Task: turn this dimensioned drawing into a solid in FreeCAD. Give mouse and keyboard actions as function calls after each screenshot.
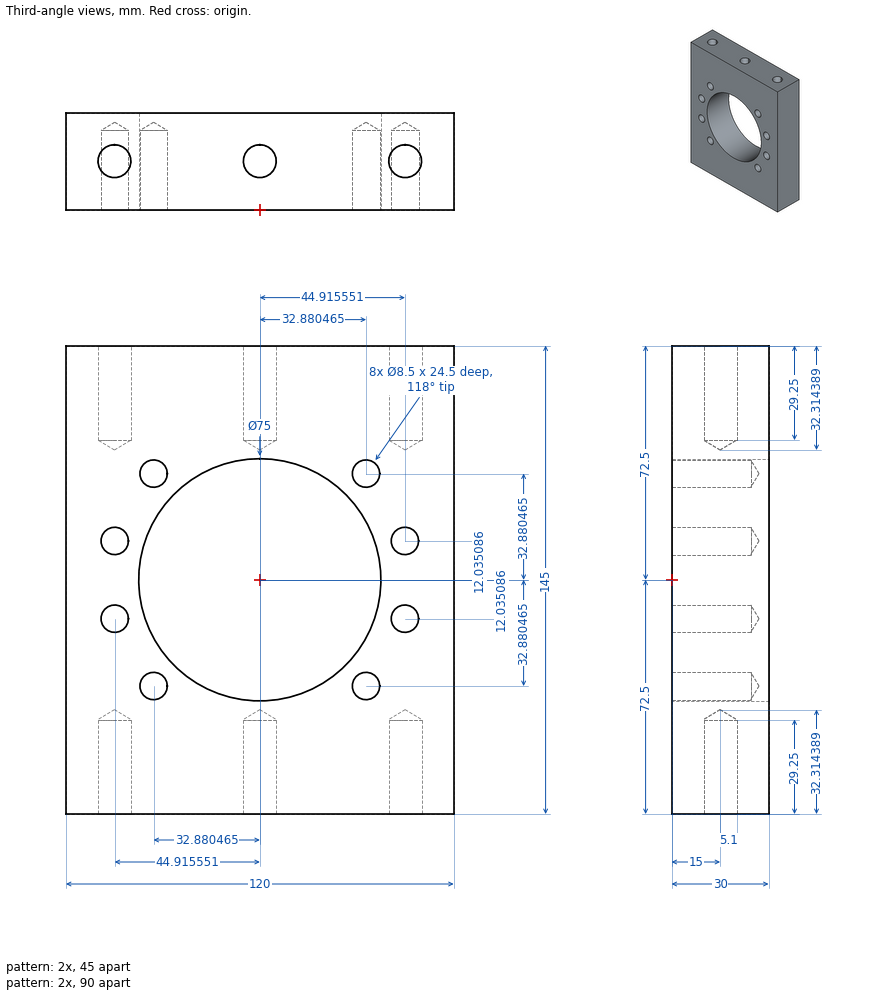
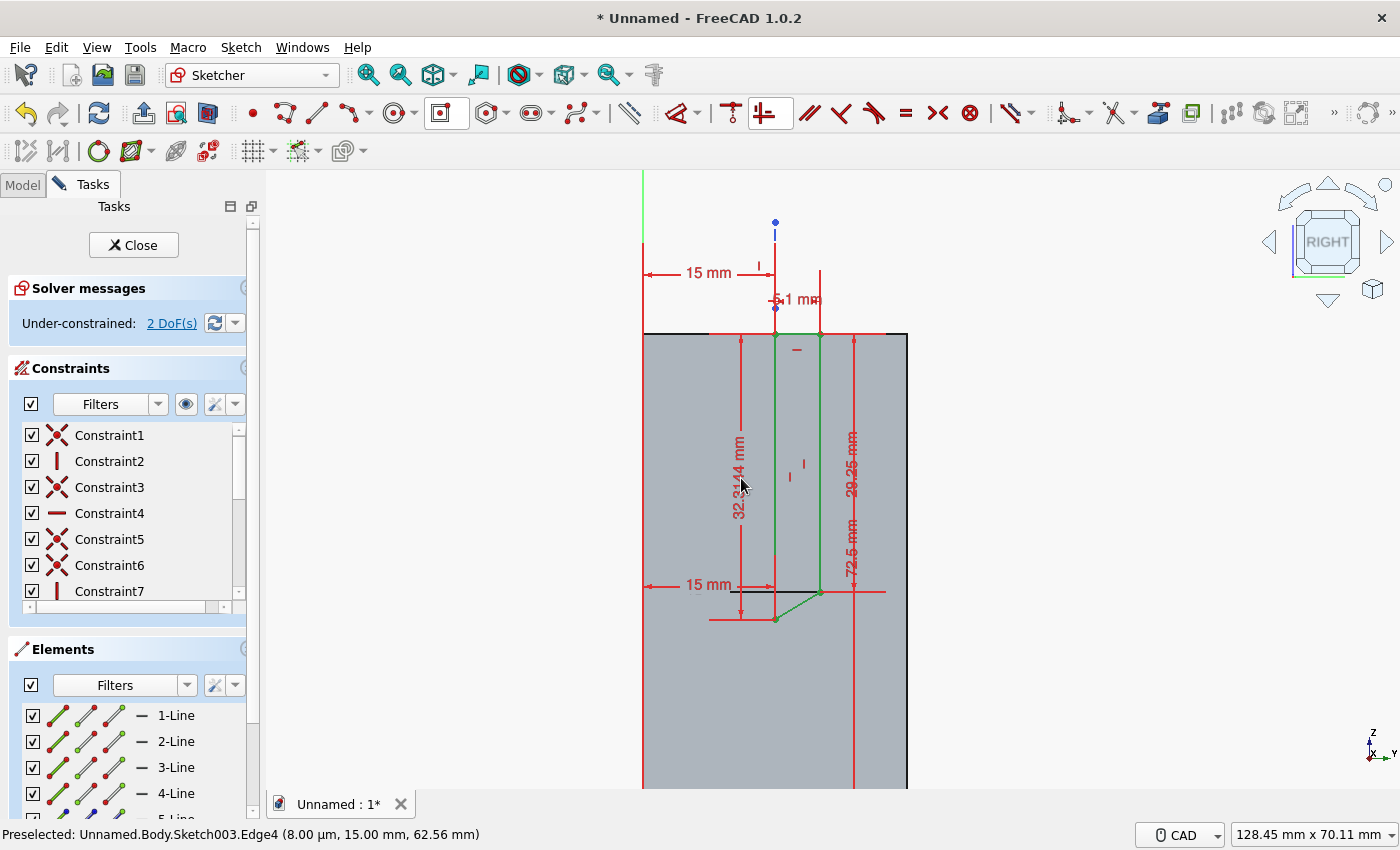
click(134, 245)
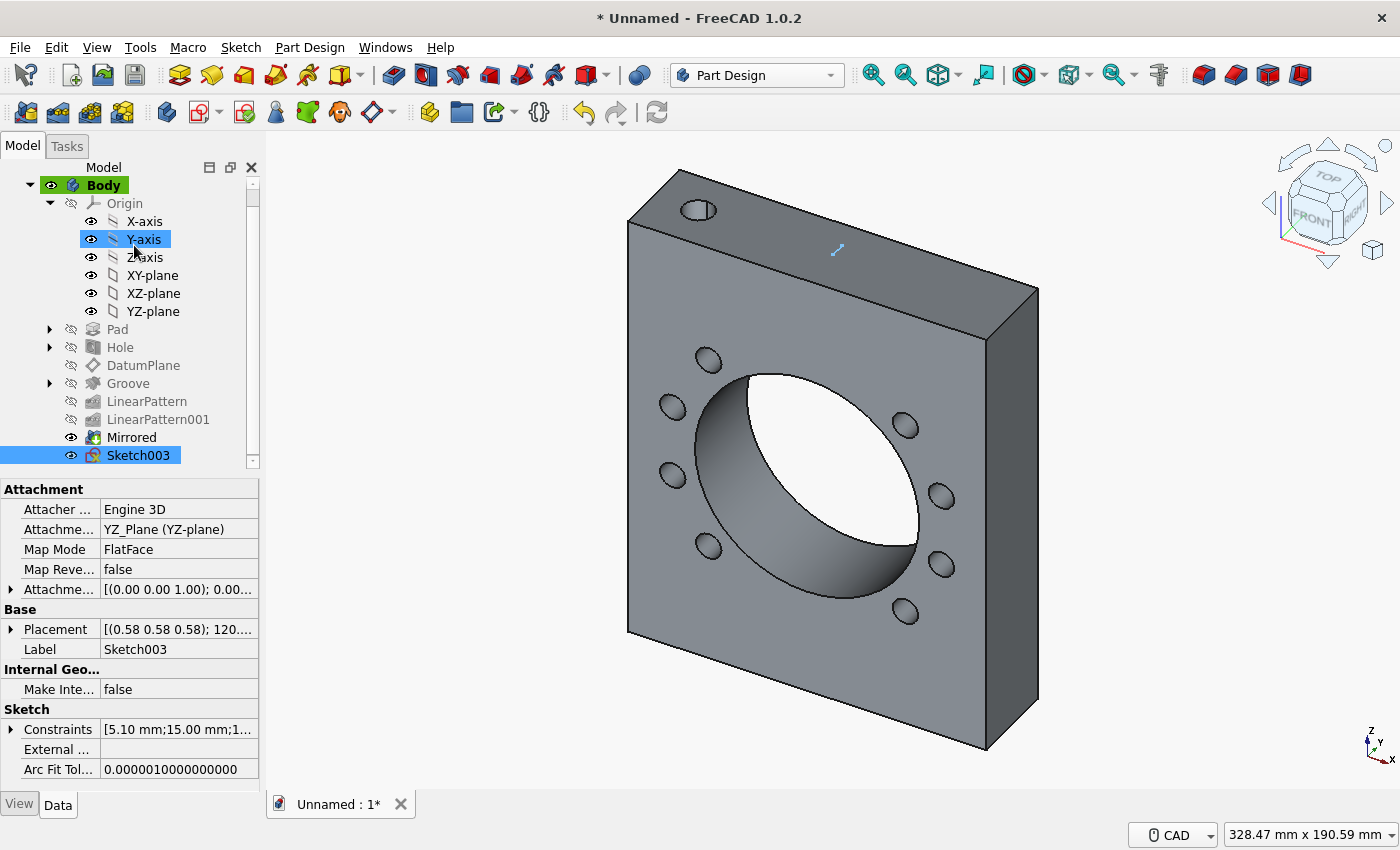
click(458, 76)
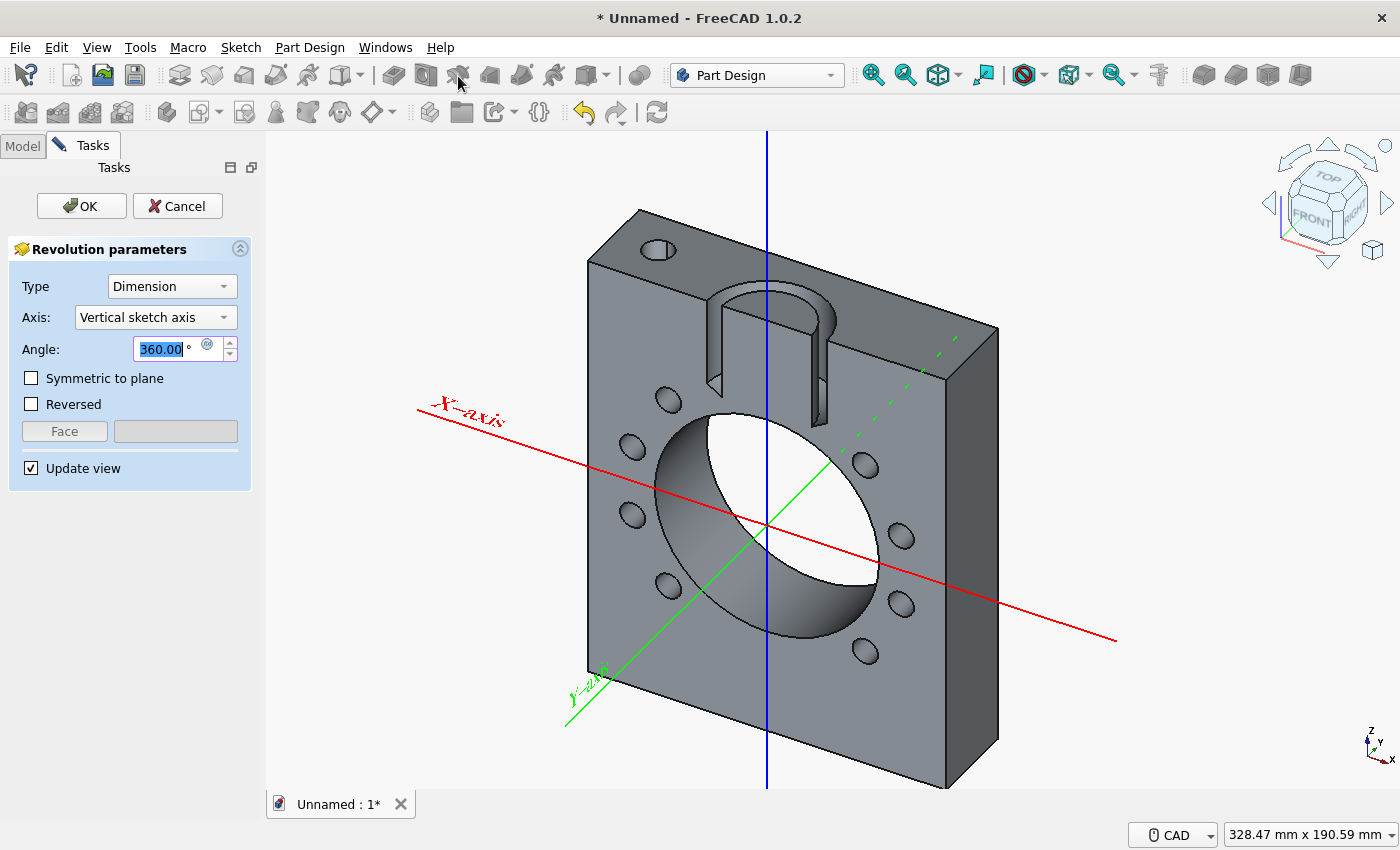
click(156, 318)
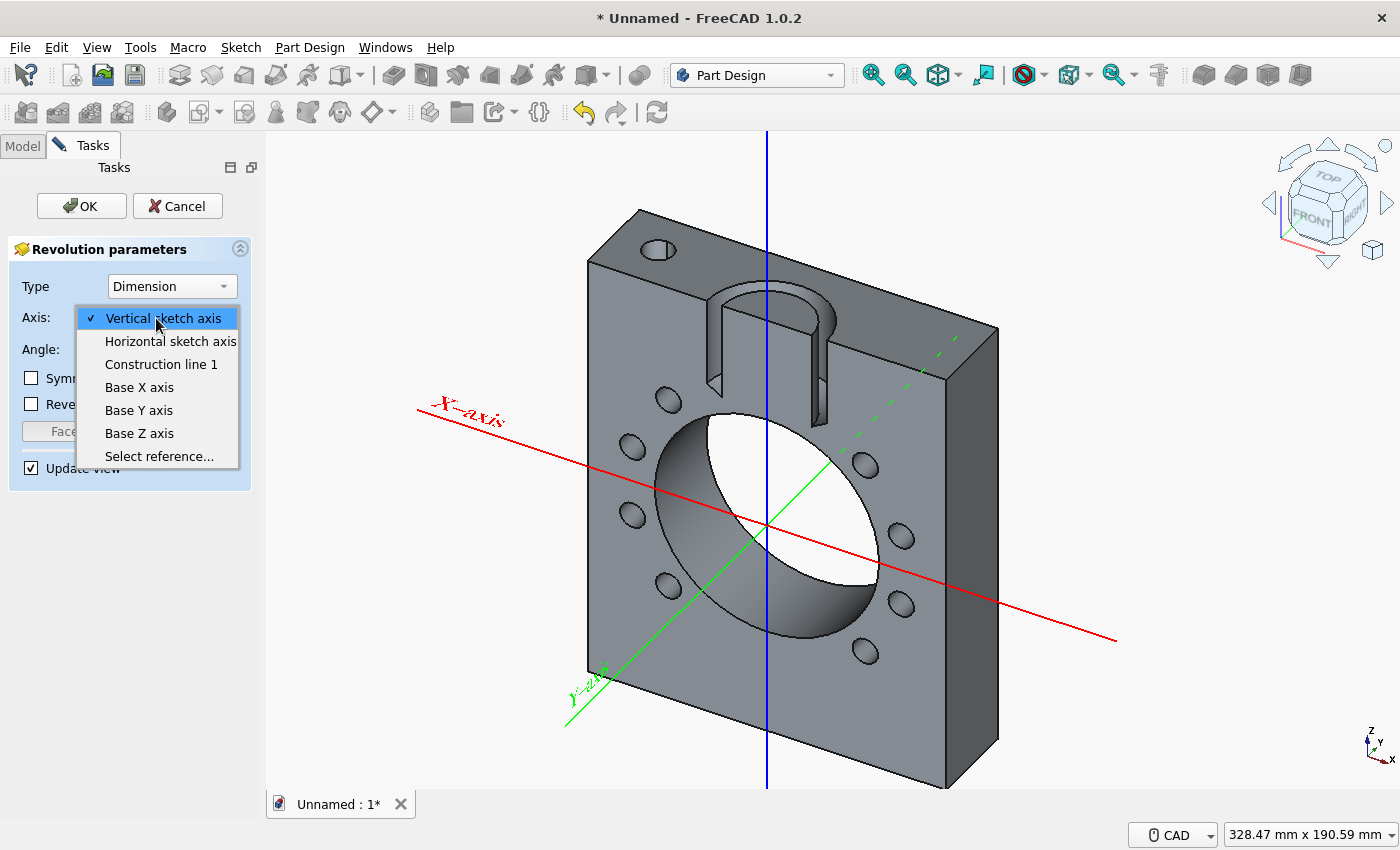
click(156, 364)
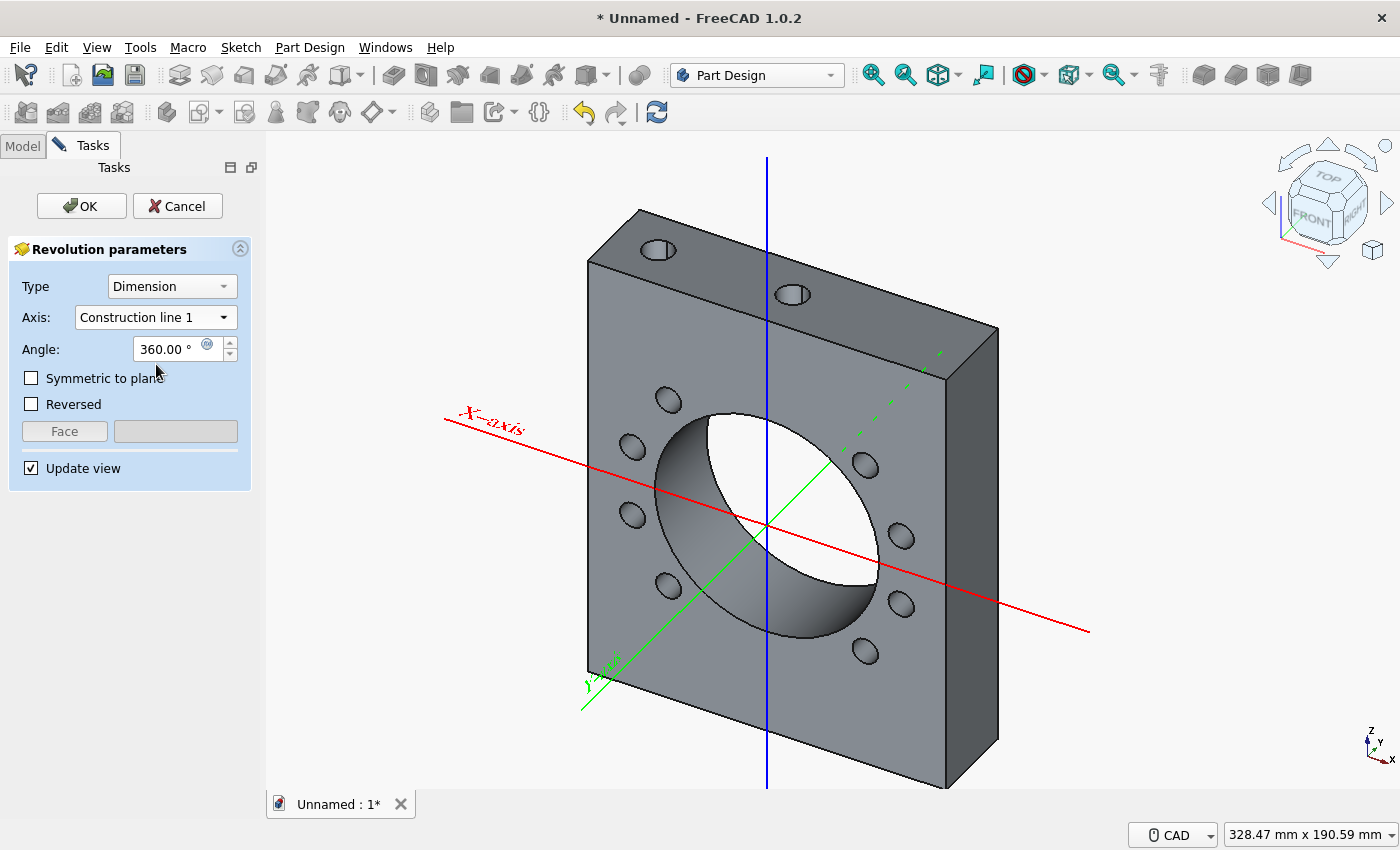
click(82, 206)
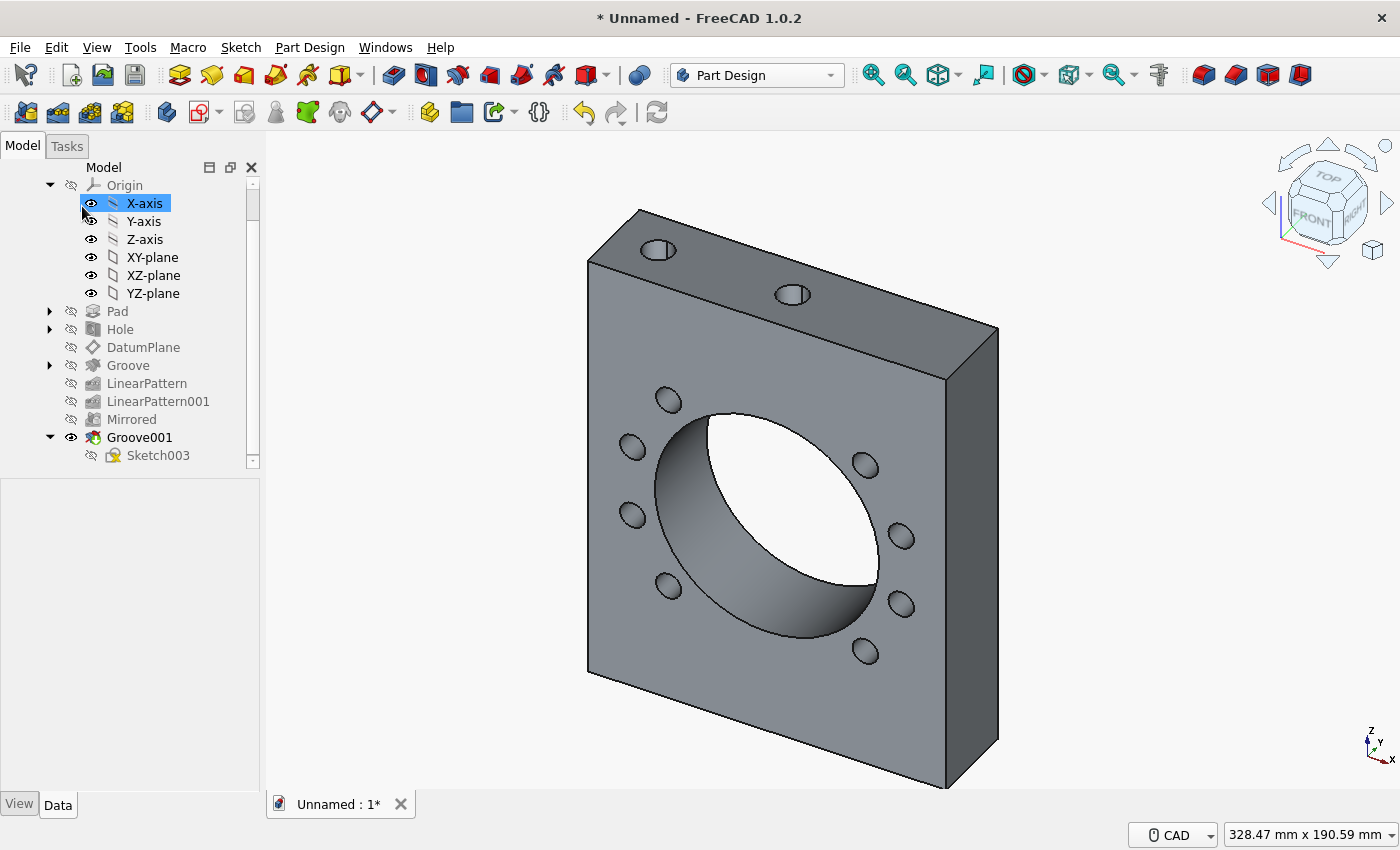
click(136, 293)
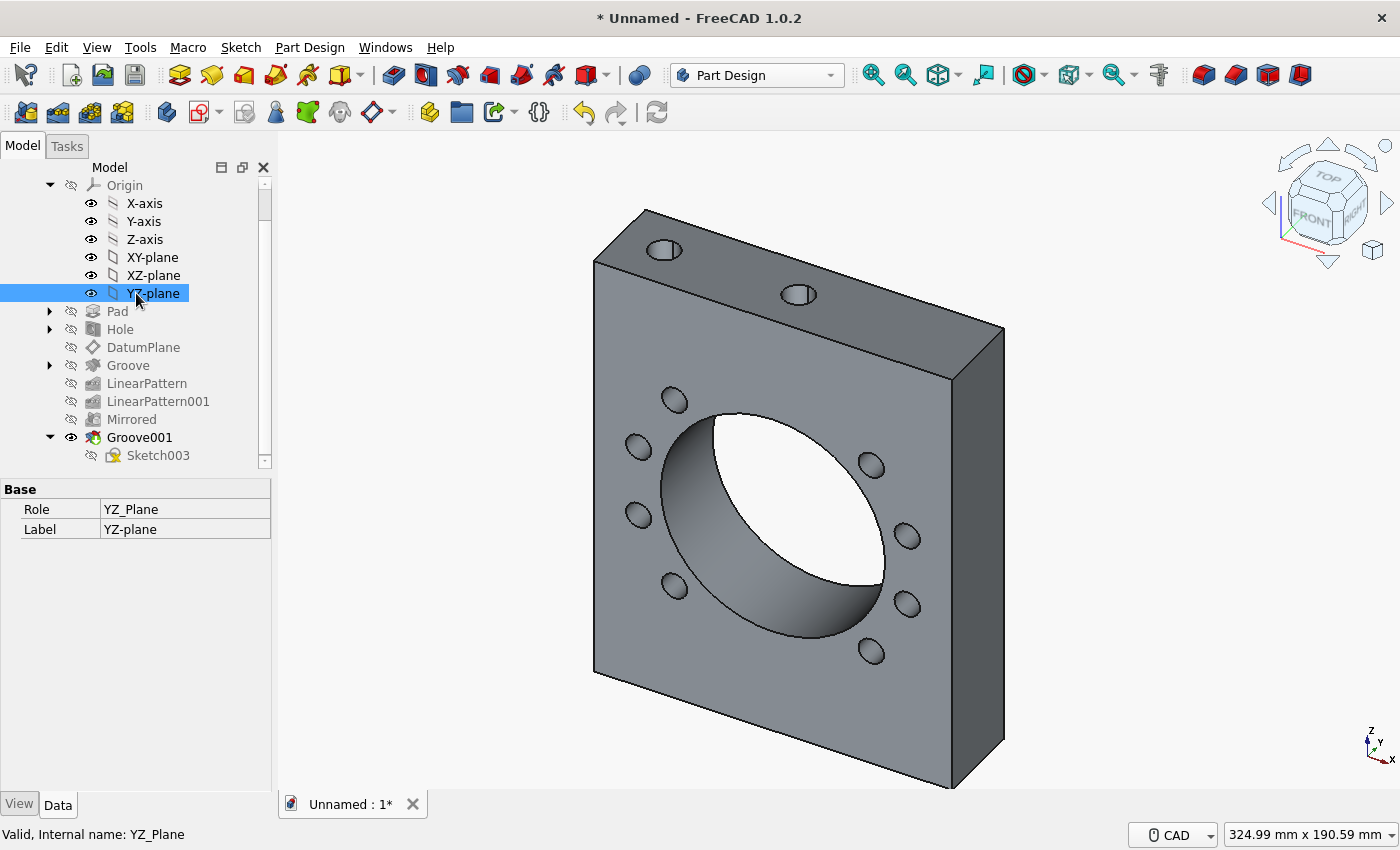
click(372, 112)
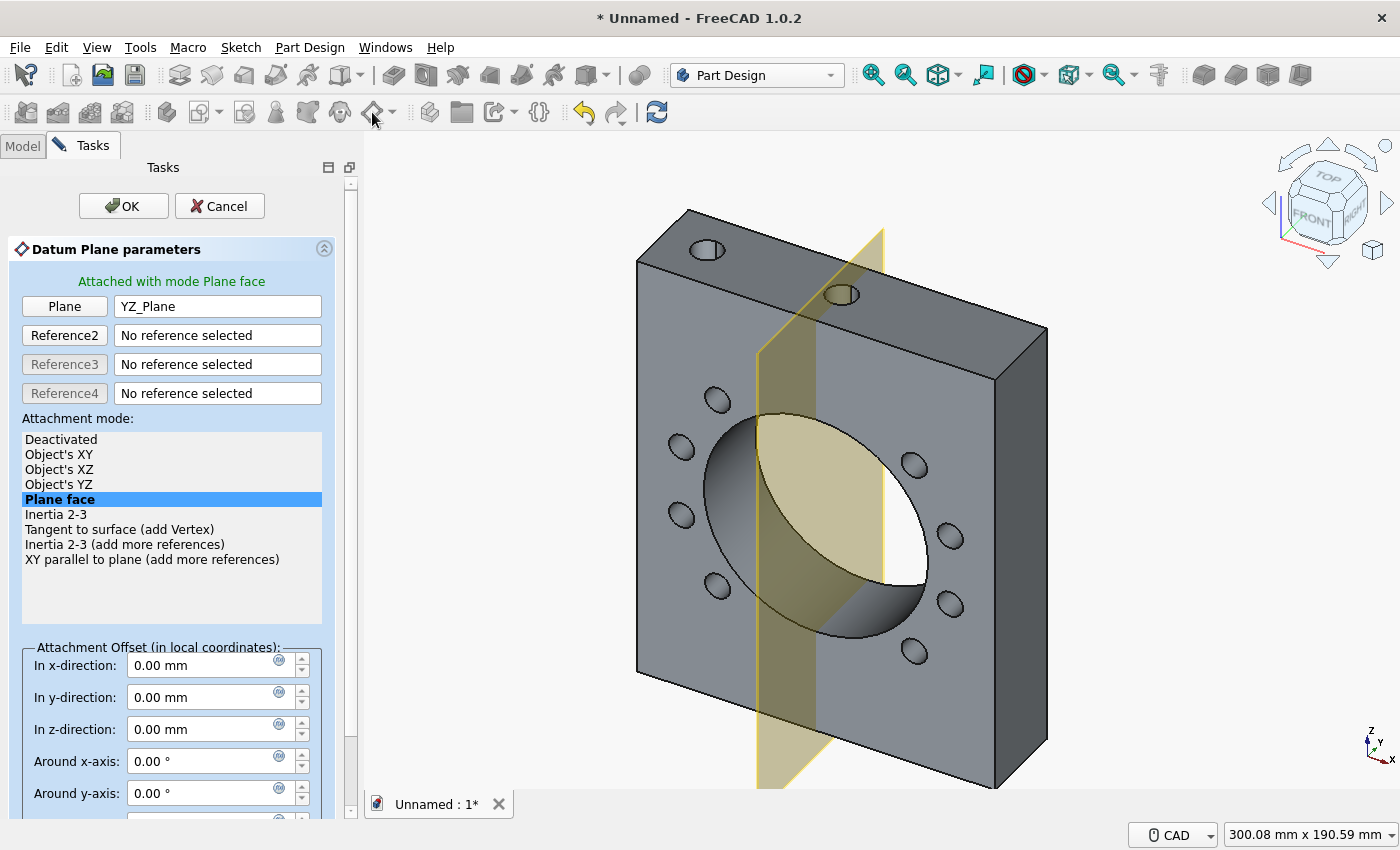
triple_click(210, 729)